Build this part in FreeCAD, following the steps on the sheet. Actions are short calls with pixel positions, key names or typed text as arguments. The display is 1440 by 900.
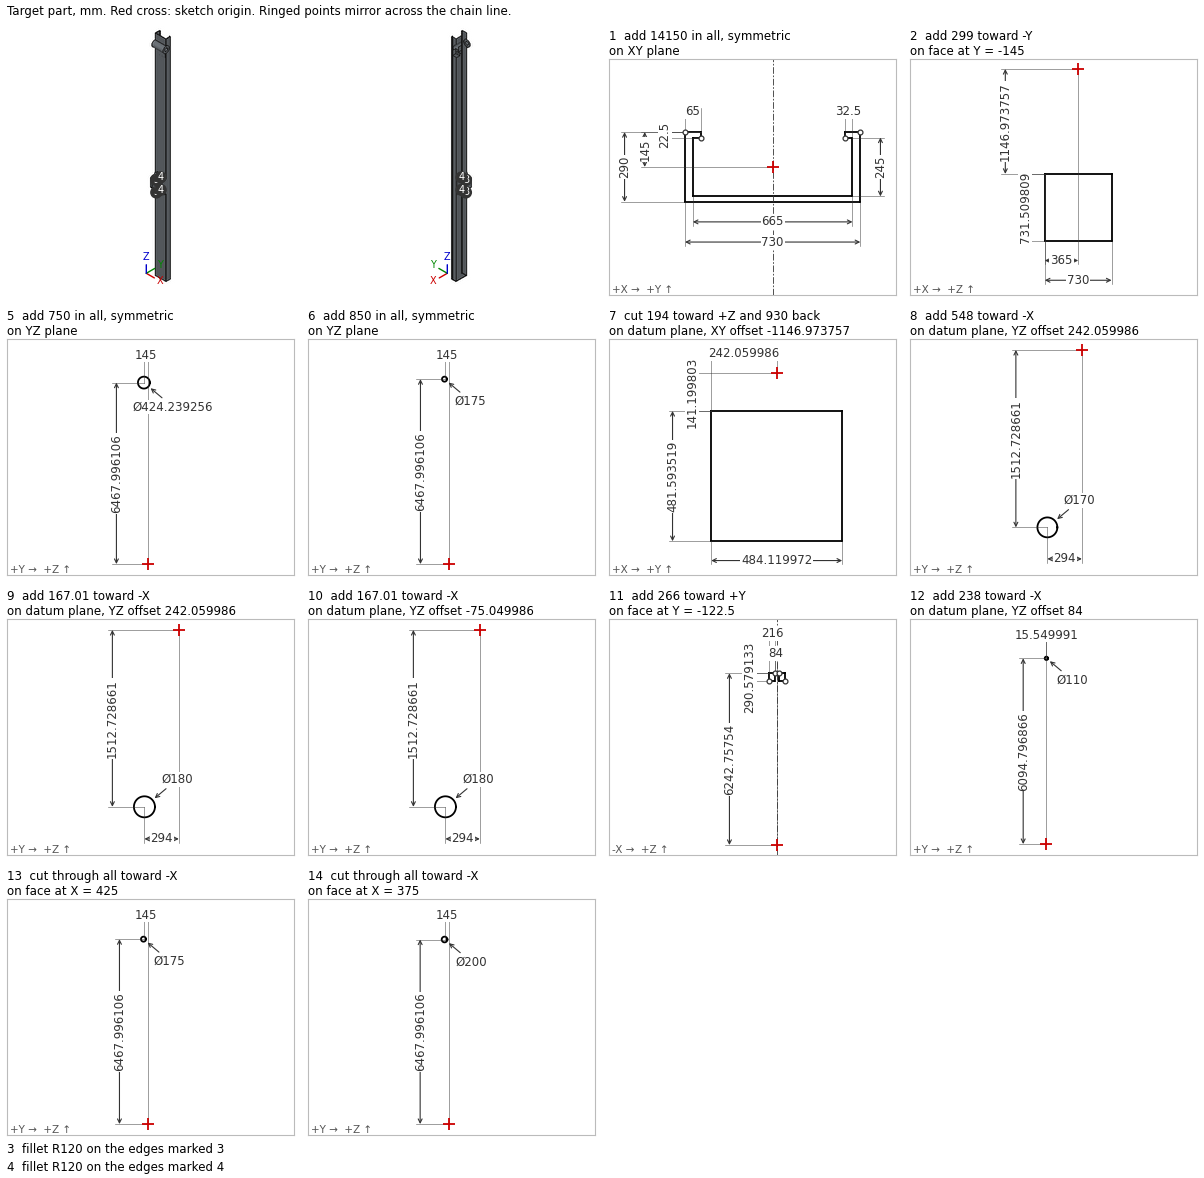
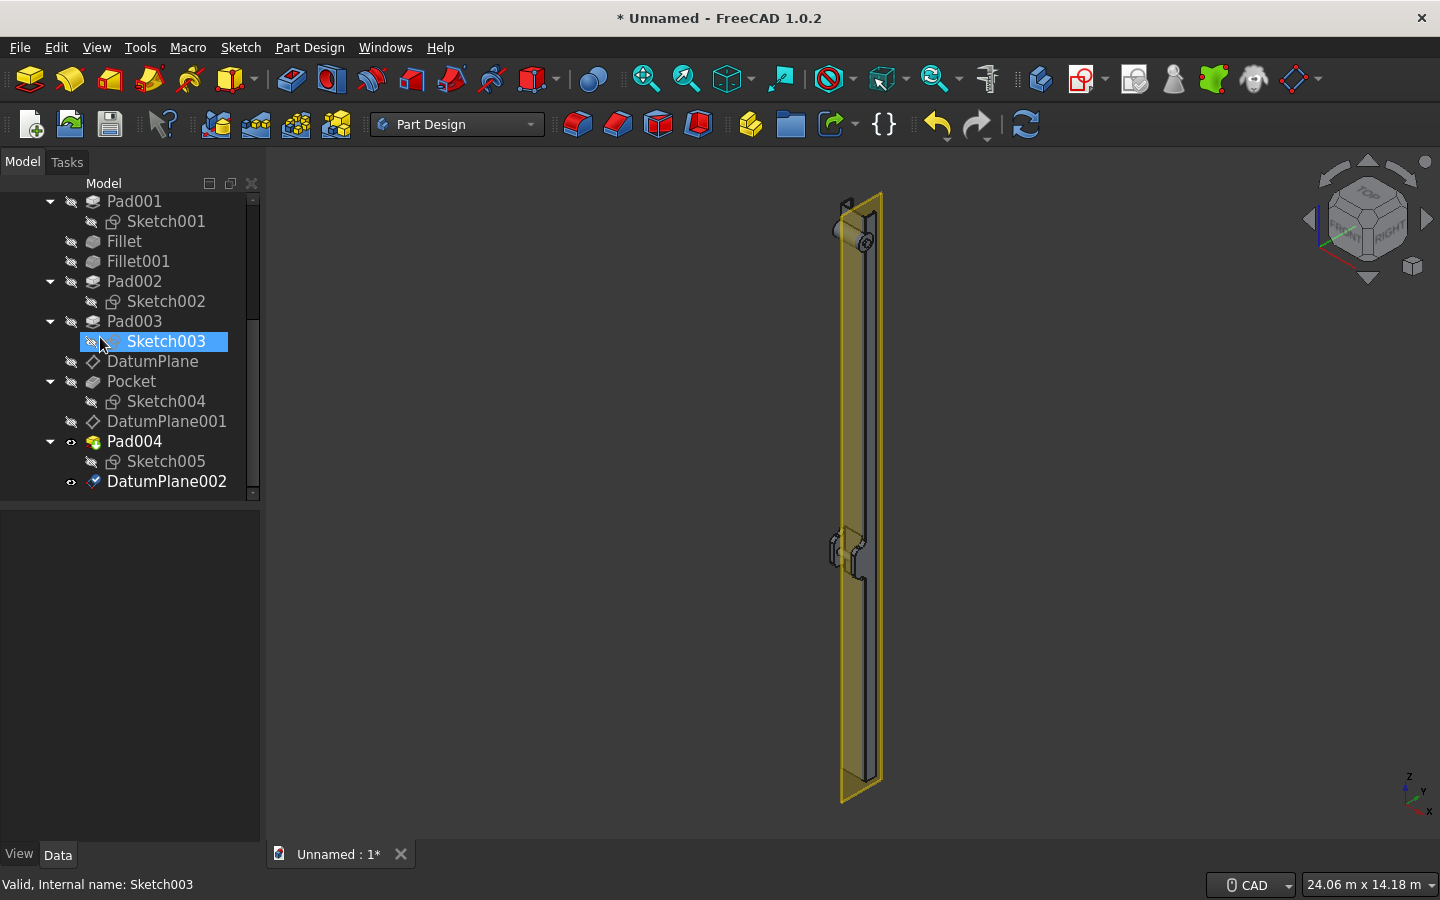
click(116, 482)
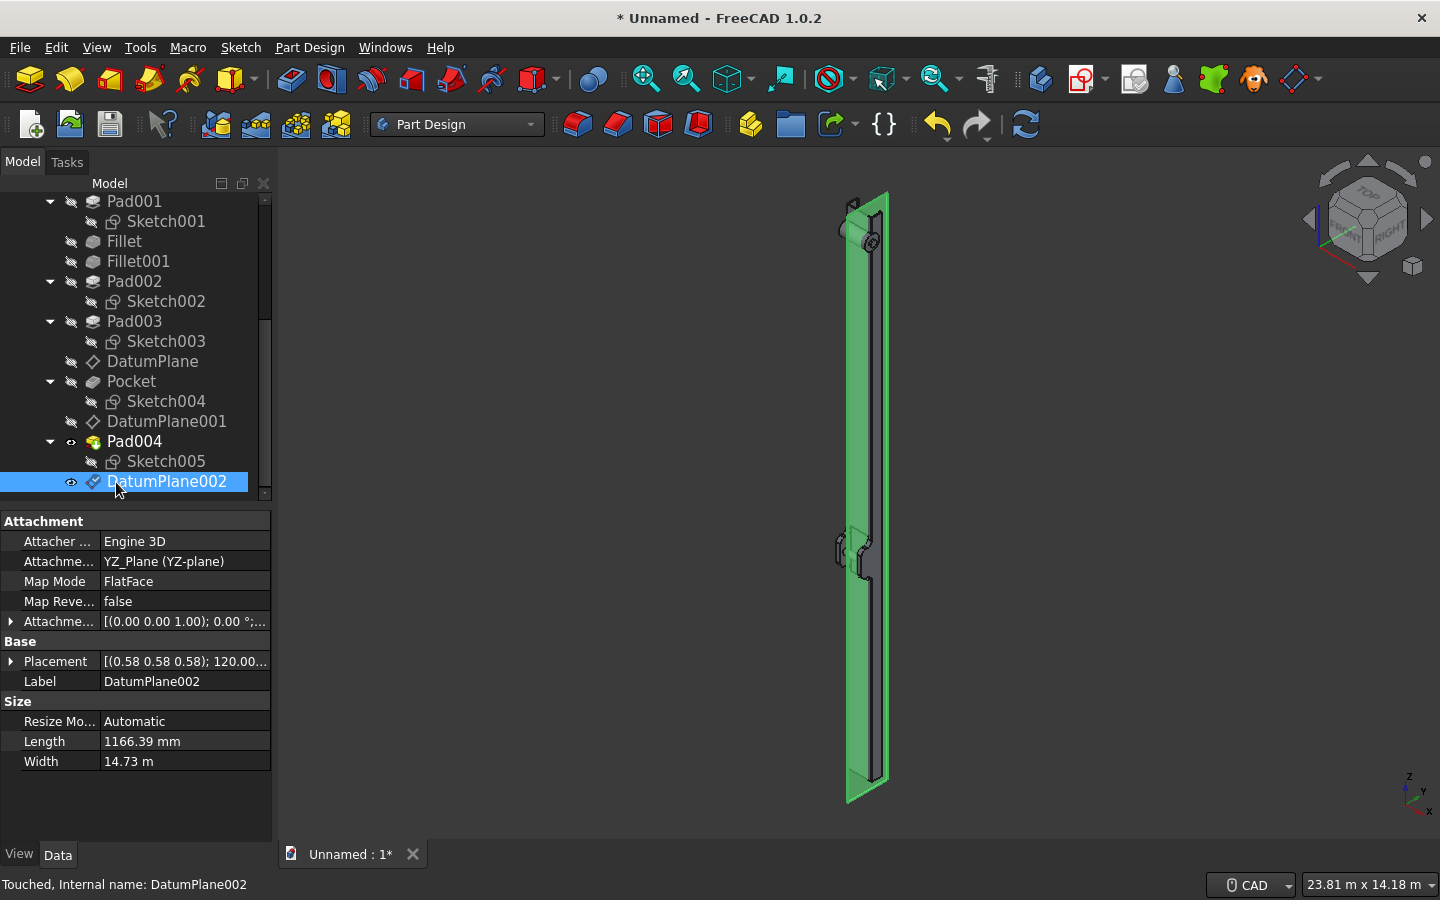
click(1082, 80)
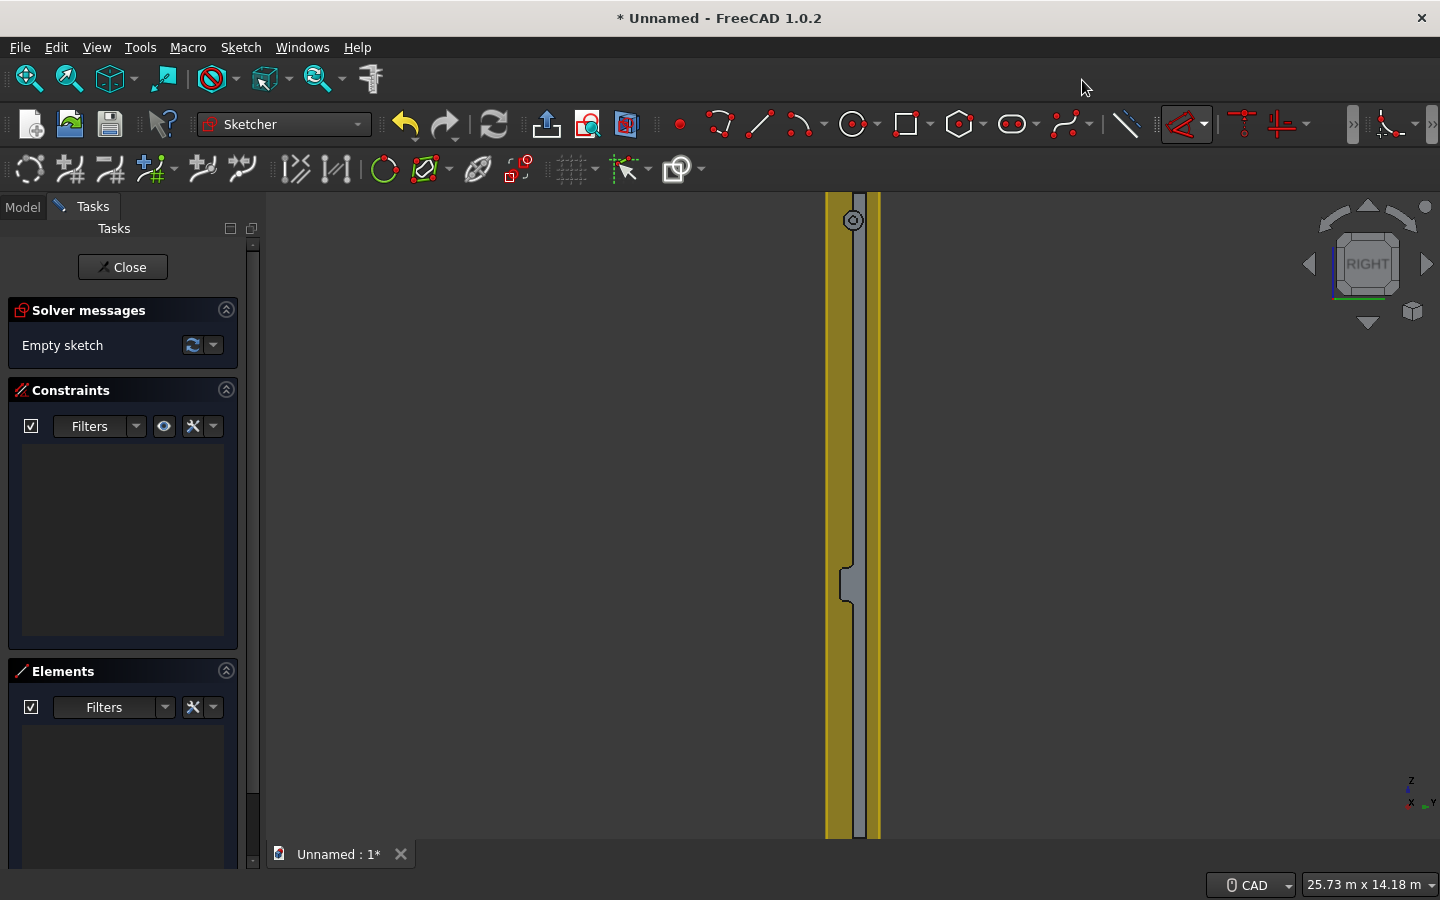
key(q)
key(s)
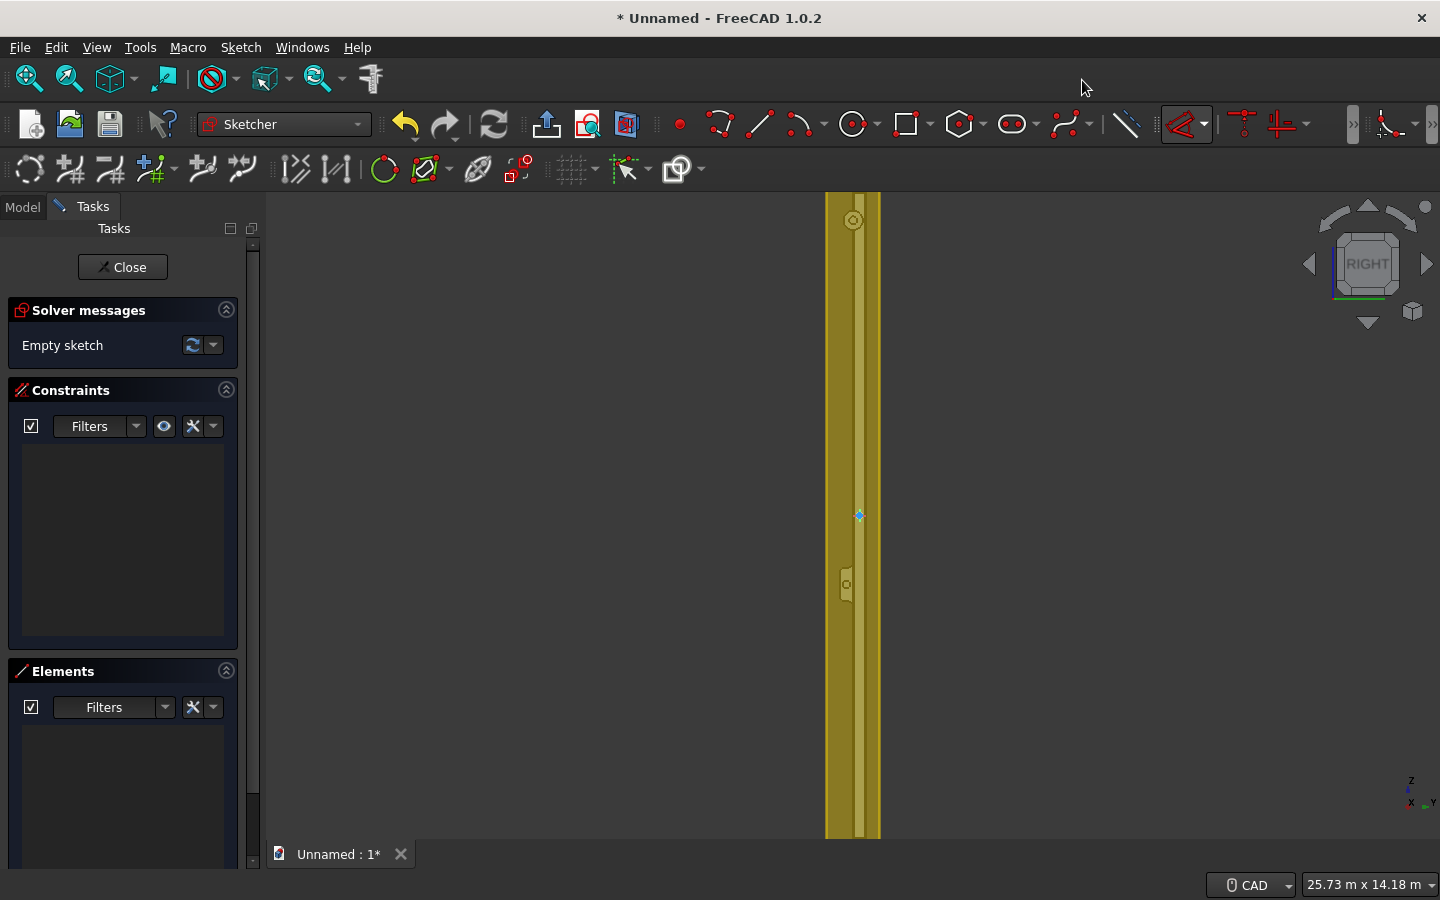
scroll(850, 588, up, 15)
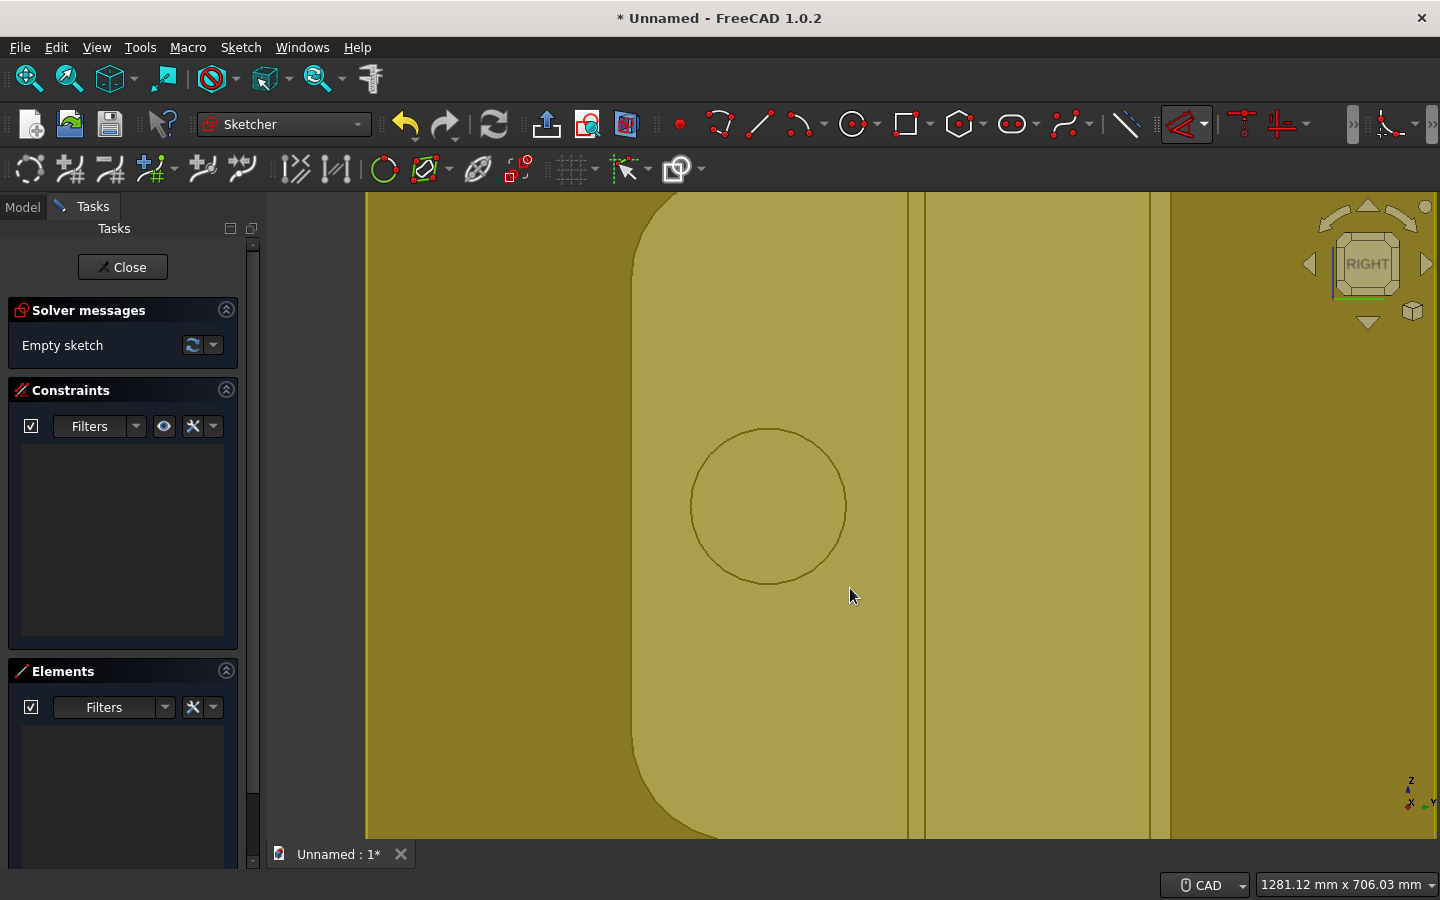
scroll(759, 501, up, 5)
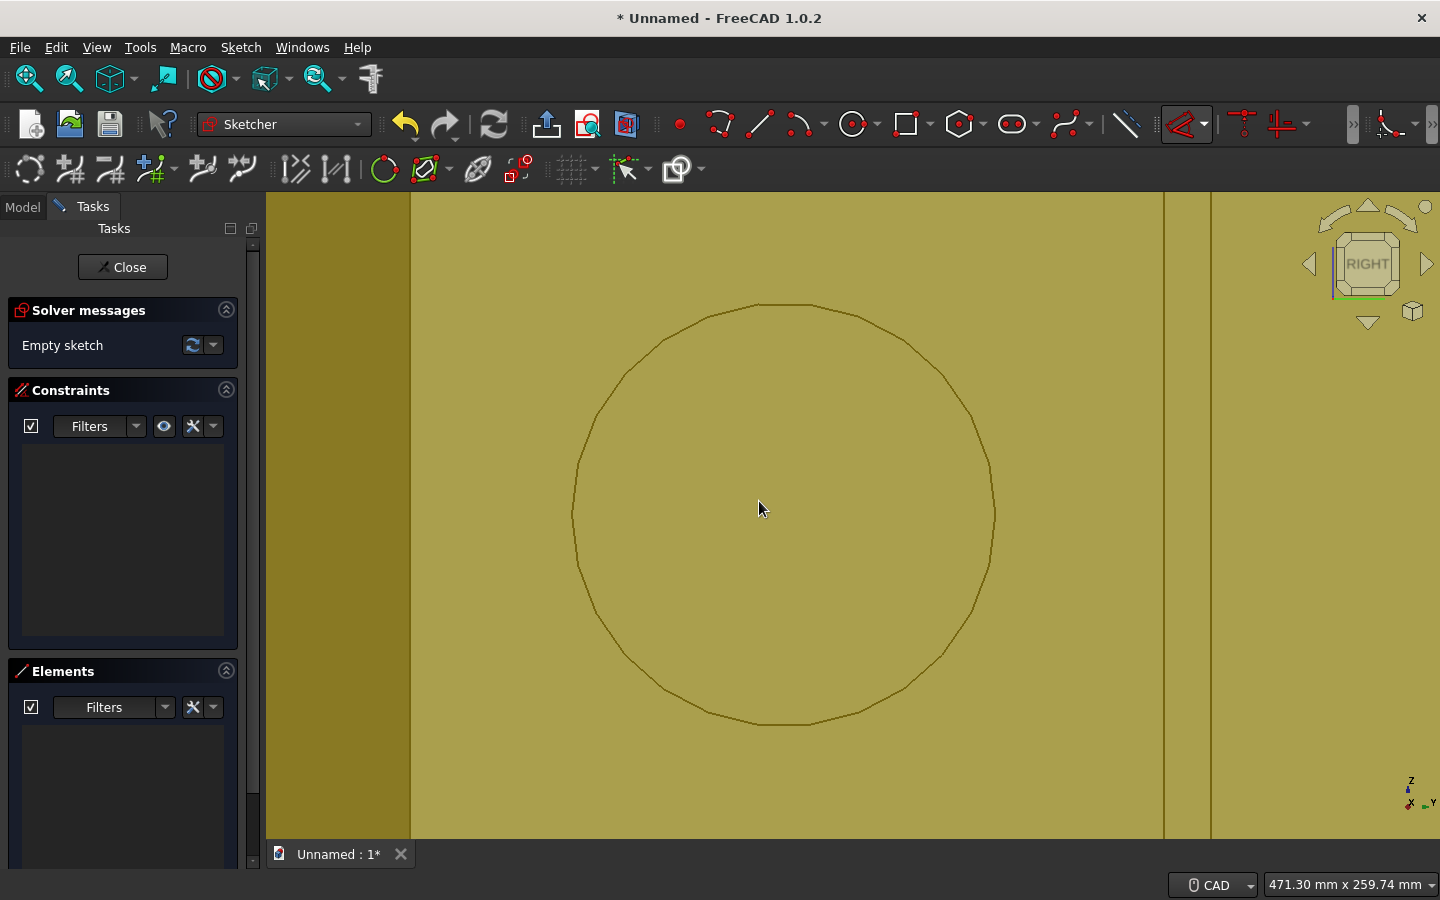
key(g)
key(c)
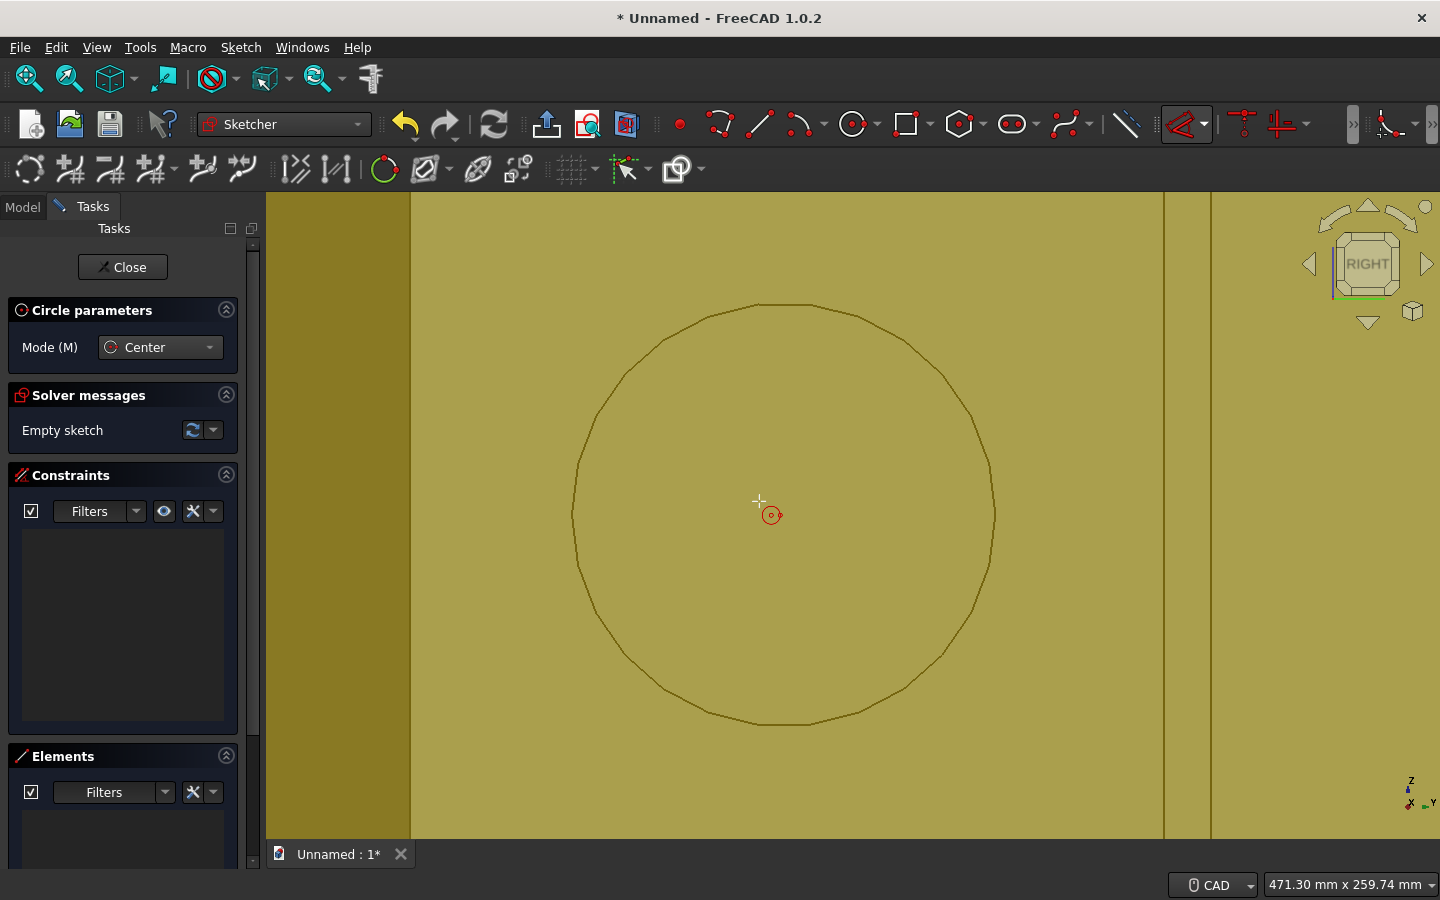
click(784, 515)
click(942, 356)
key(Escape)